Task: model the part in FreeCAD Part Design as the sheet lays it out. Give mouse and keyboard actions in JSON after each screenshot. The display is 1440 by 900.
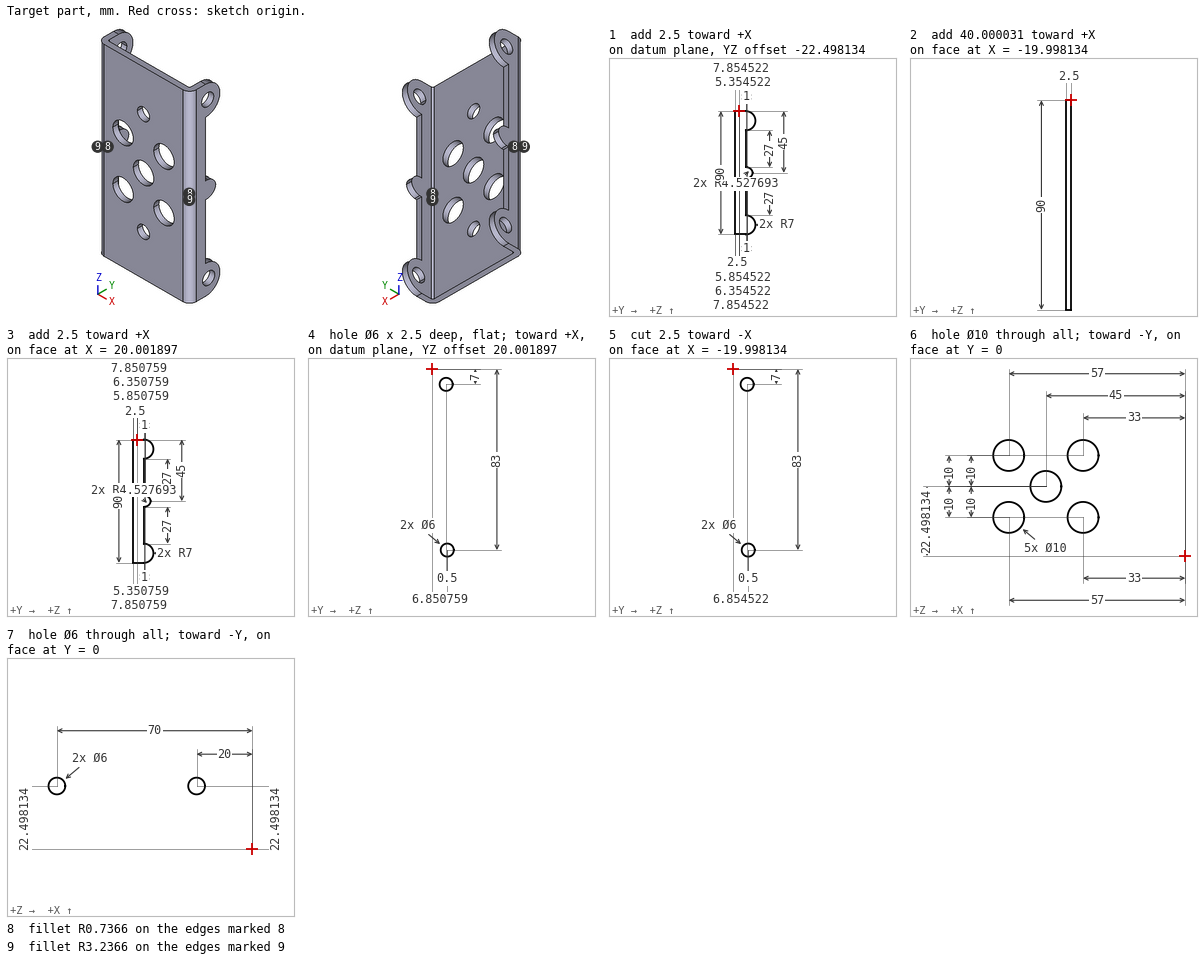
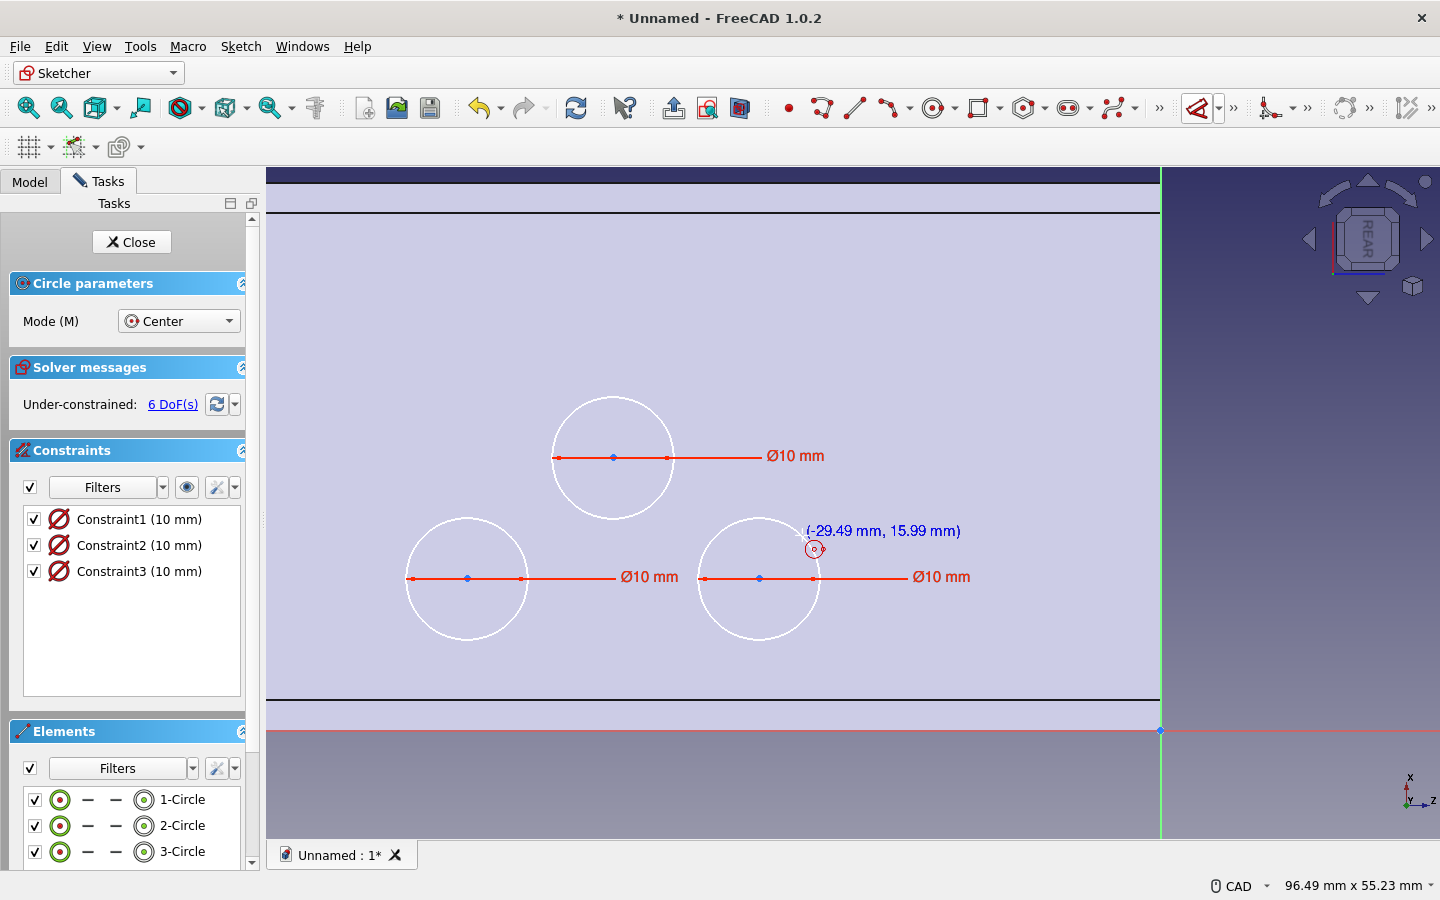
{"action": "left_click", "coordinate": [759, 335]}
{"action": "mouse_move", "coordinate": [802, 292]}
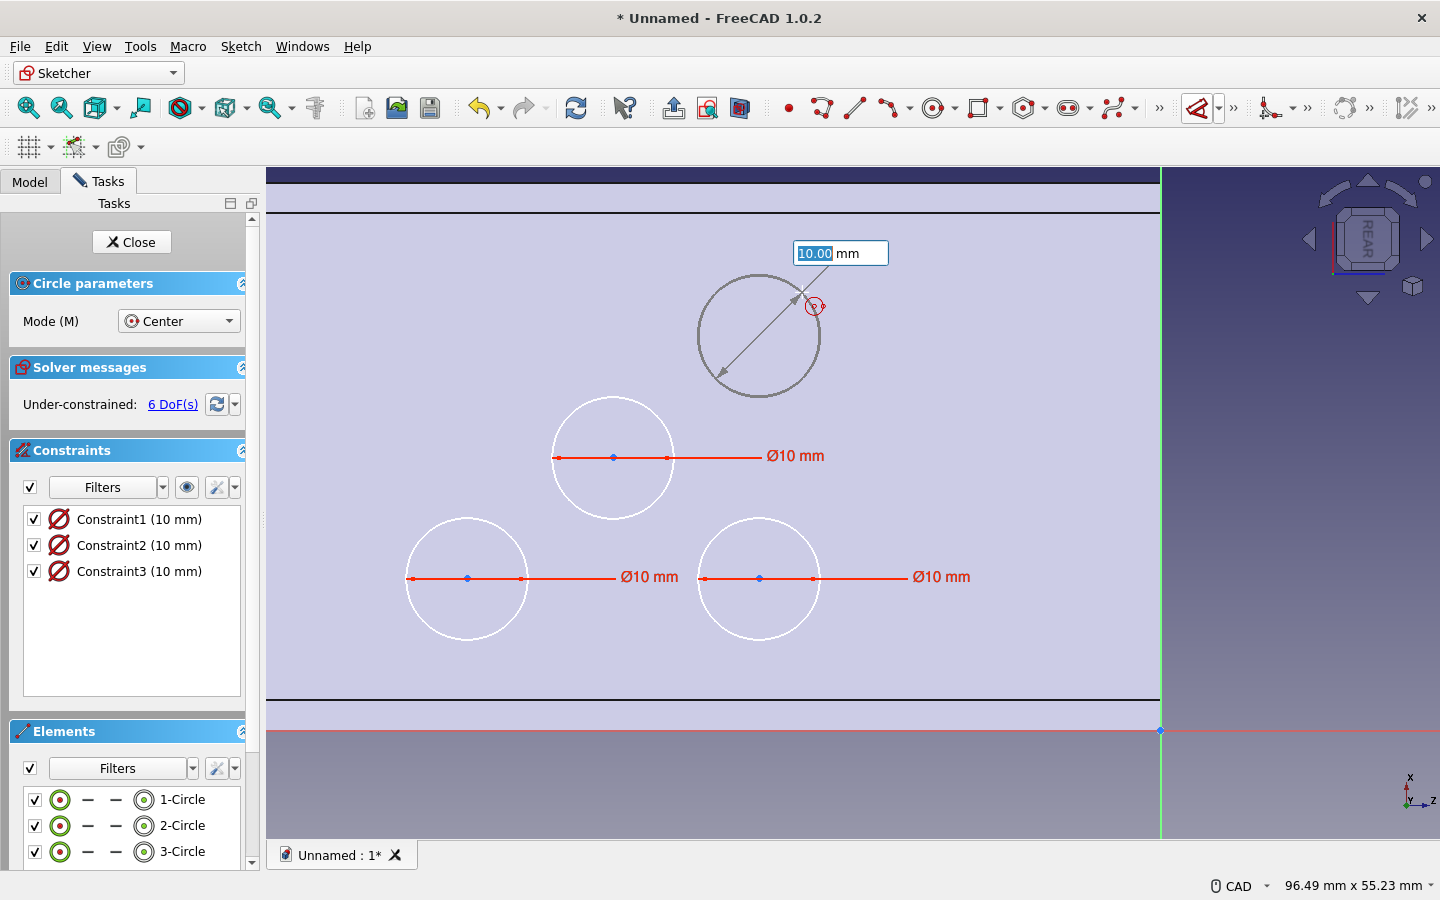
{"action": "type", "text": "10"}
{"action": "key", "text": "Return"}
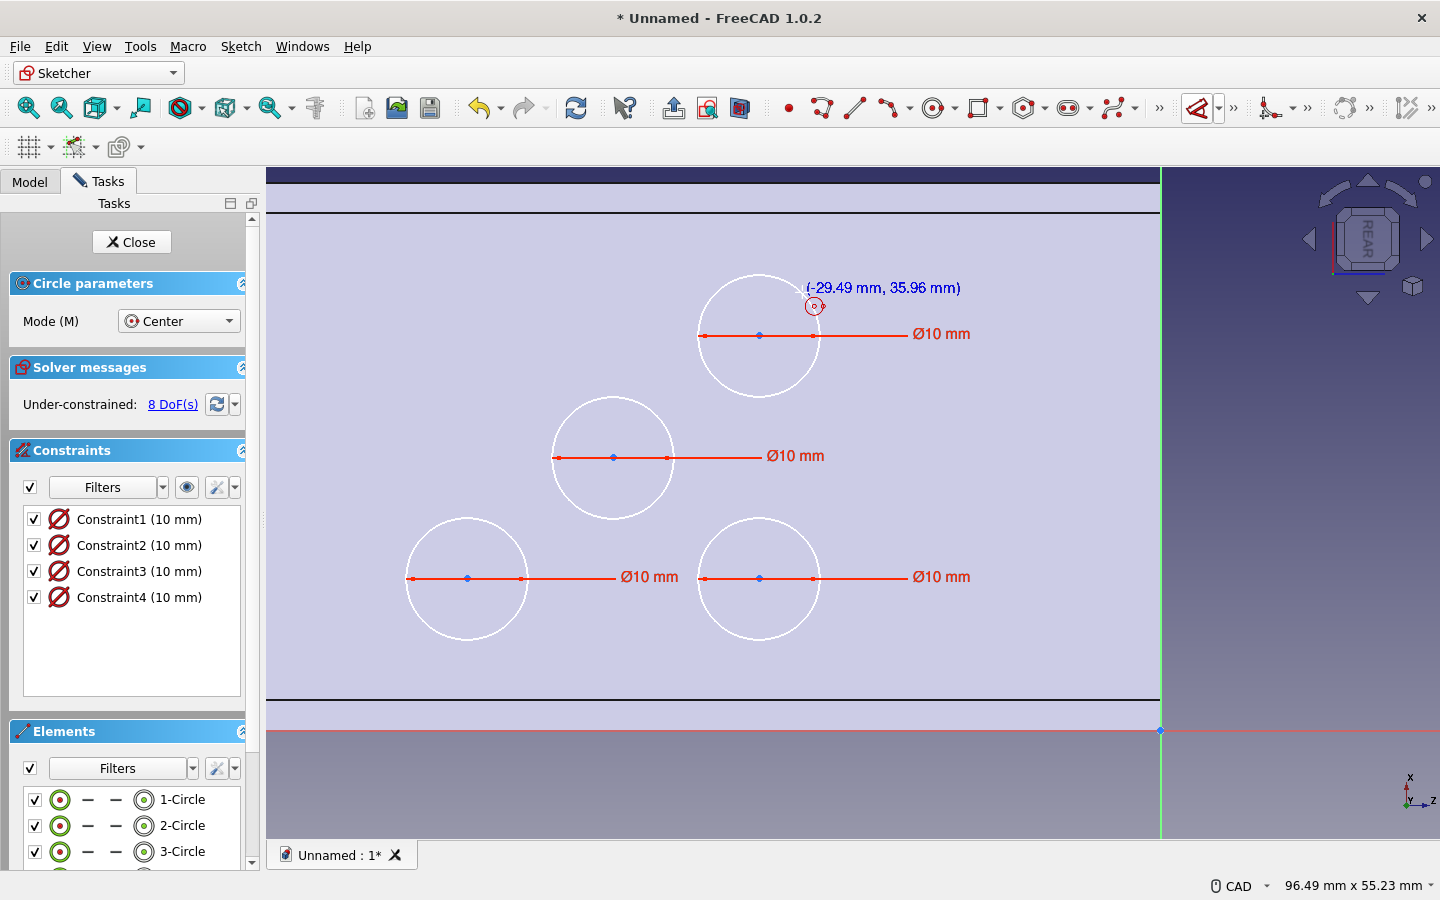
{"action": "left_click", "coordinate": [467, 335]}
{"action": "mouse_move", "coordinate": [510, 292]}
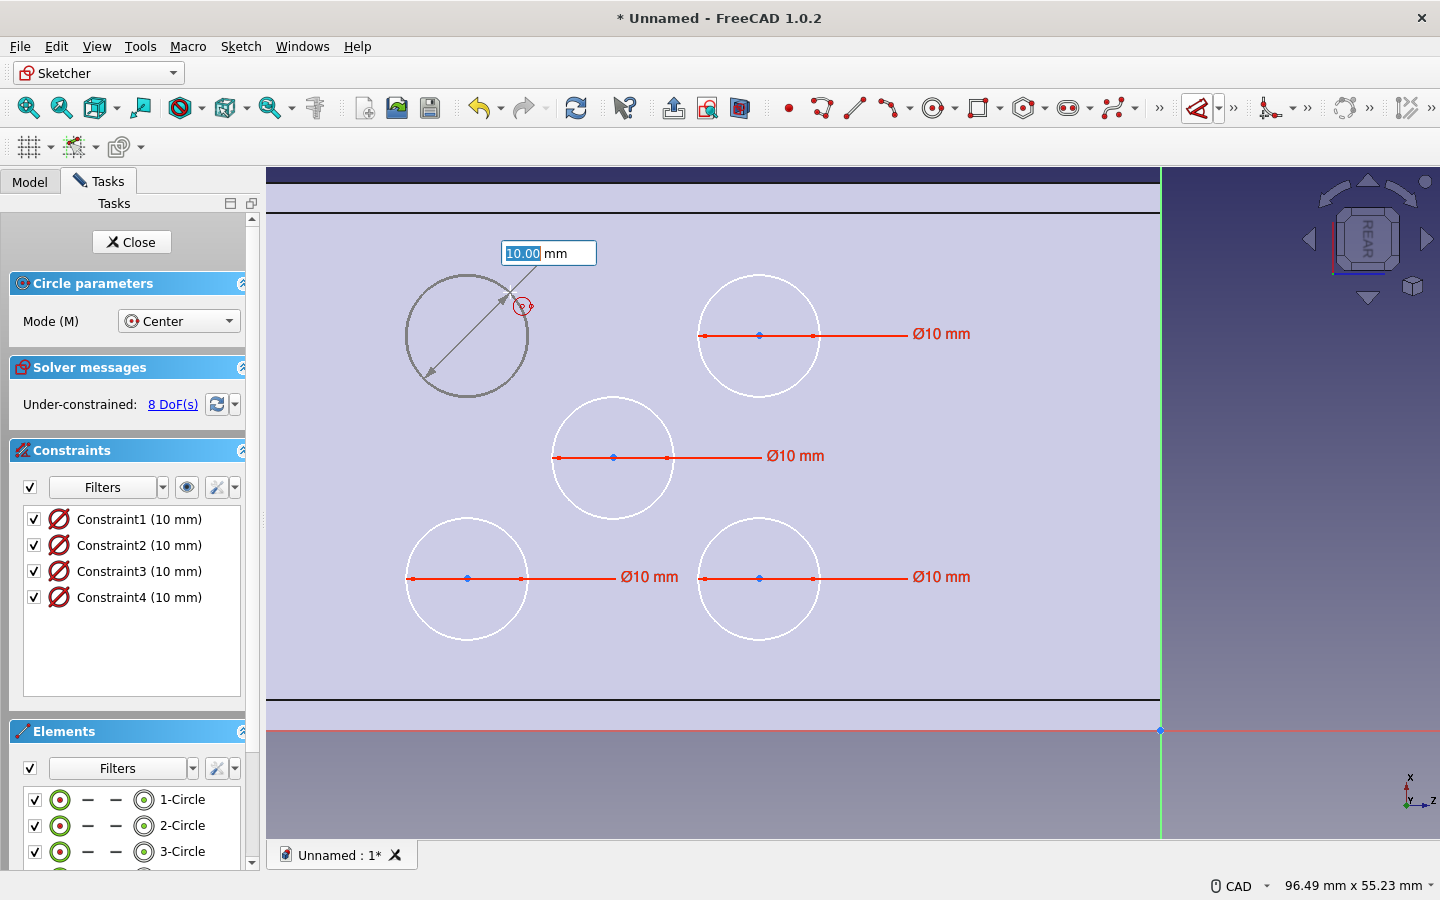
{"action": "type", "text": "10"}
{"action": "key", "text": "Return"}
{"action": "key", "text": "Escape"}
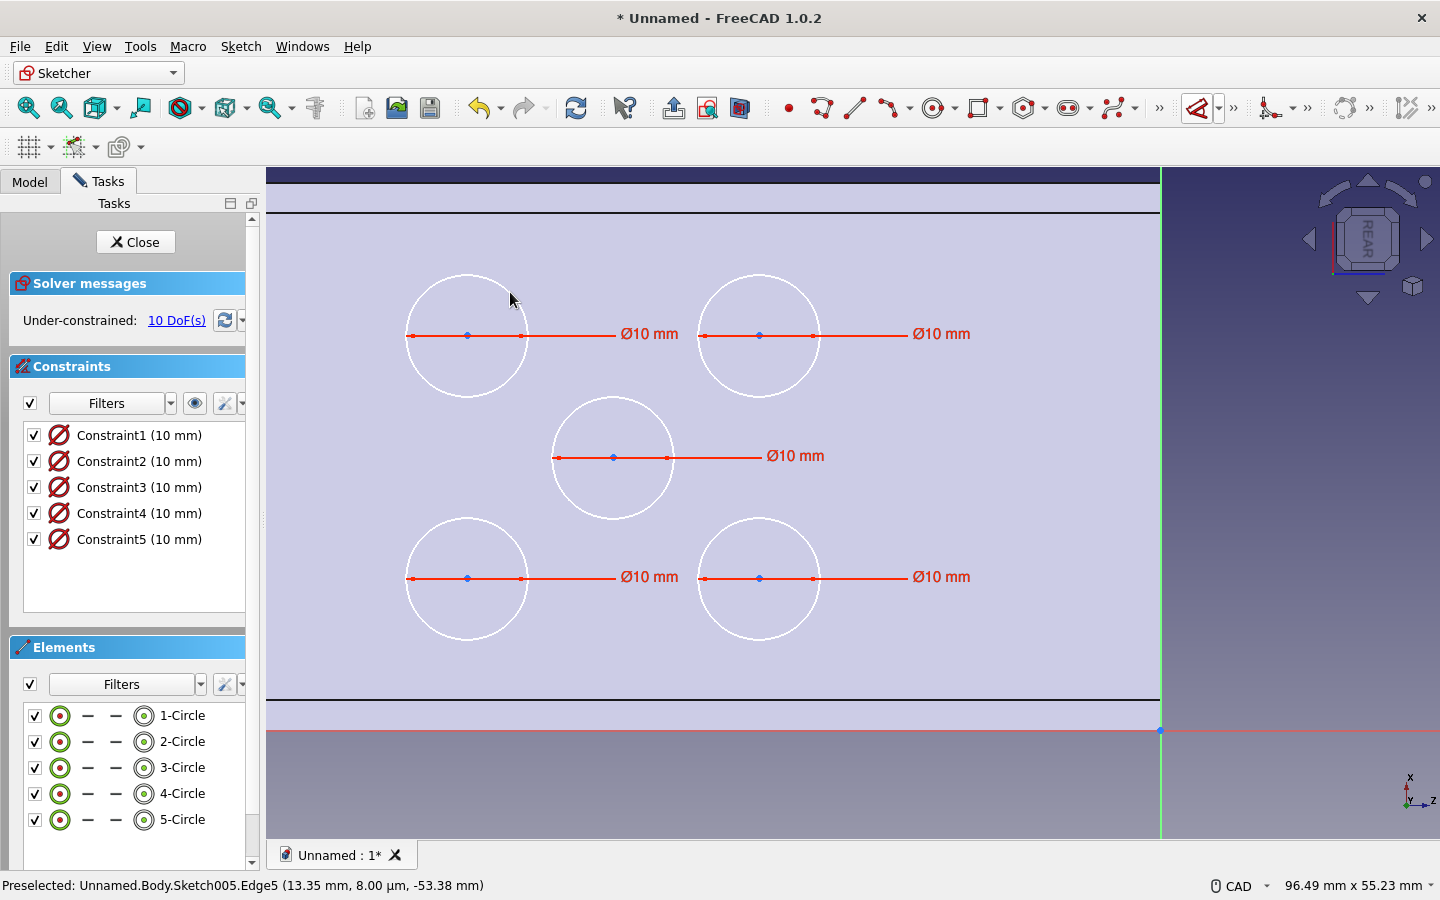
{"action": "left_click", "coordinate": [613, 458]}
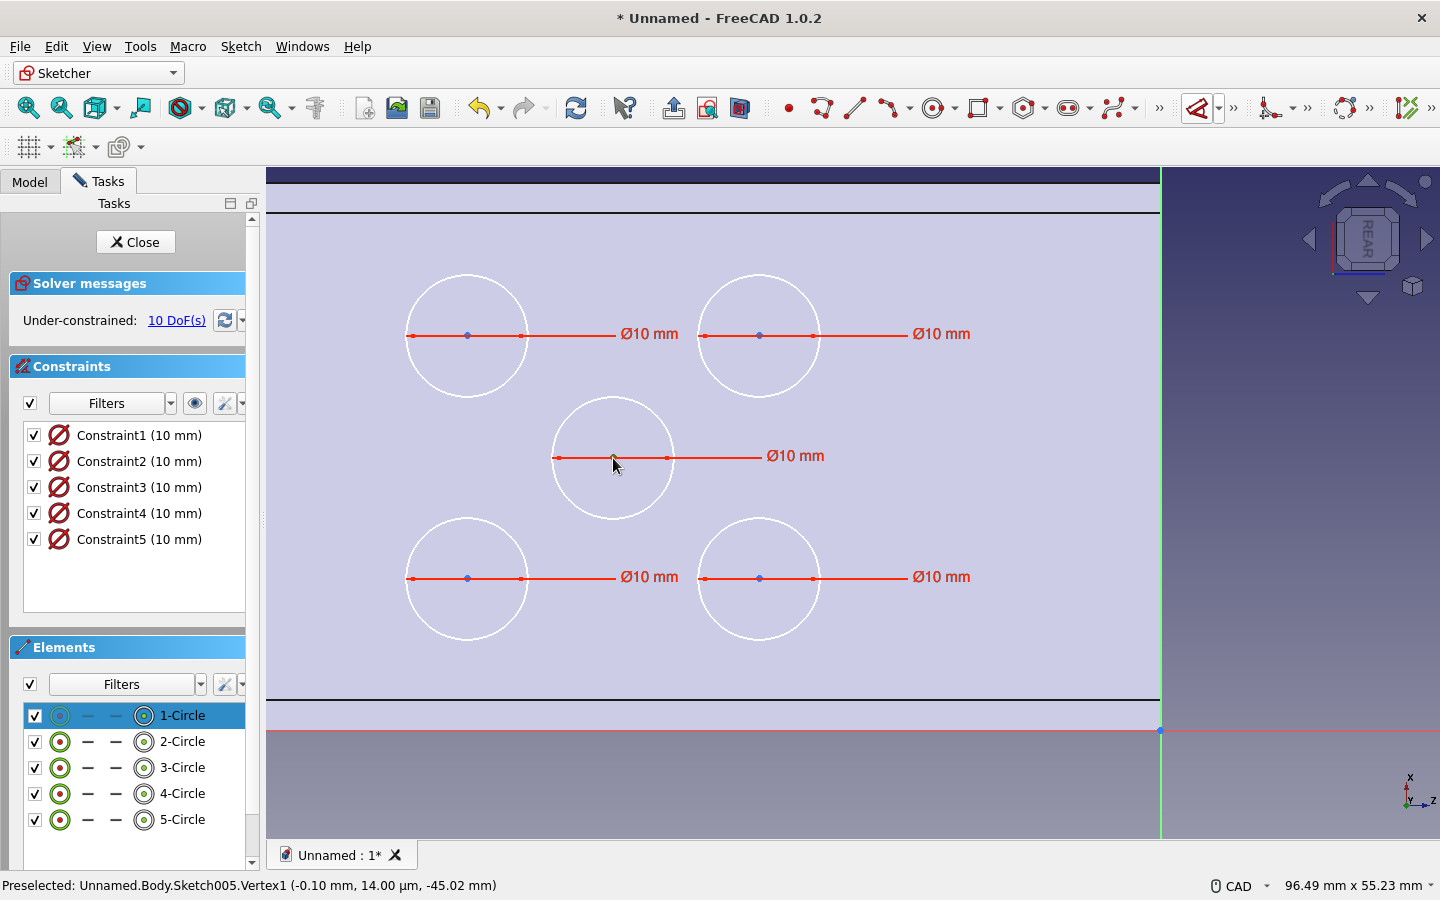
{"action": "key", "text": "l"}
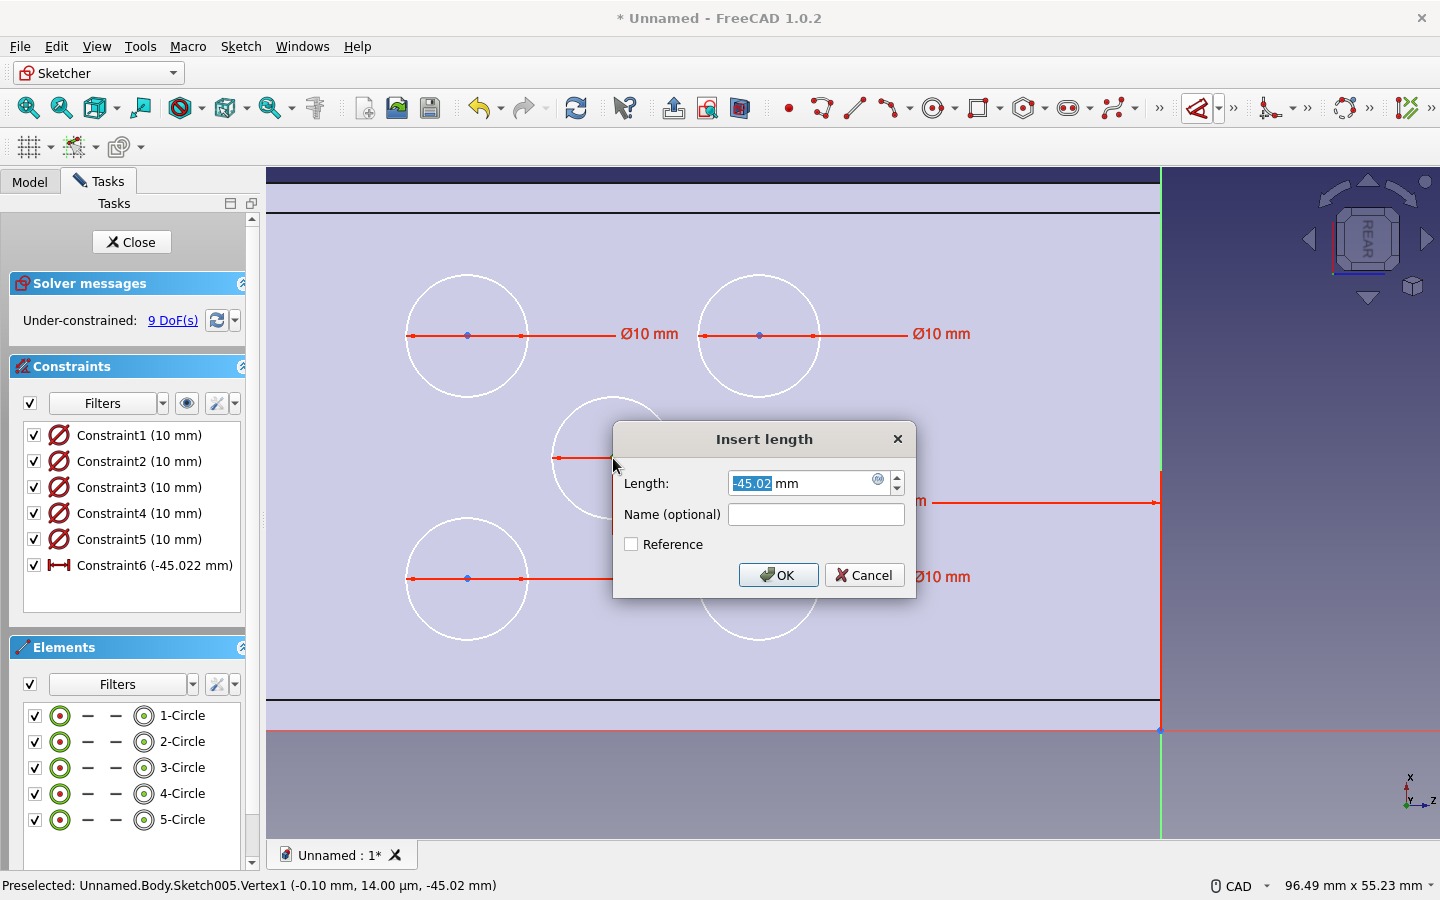
{"action": "type", "text": "-45"}
{"action": "key", "text": "Return"}